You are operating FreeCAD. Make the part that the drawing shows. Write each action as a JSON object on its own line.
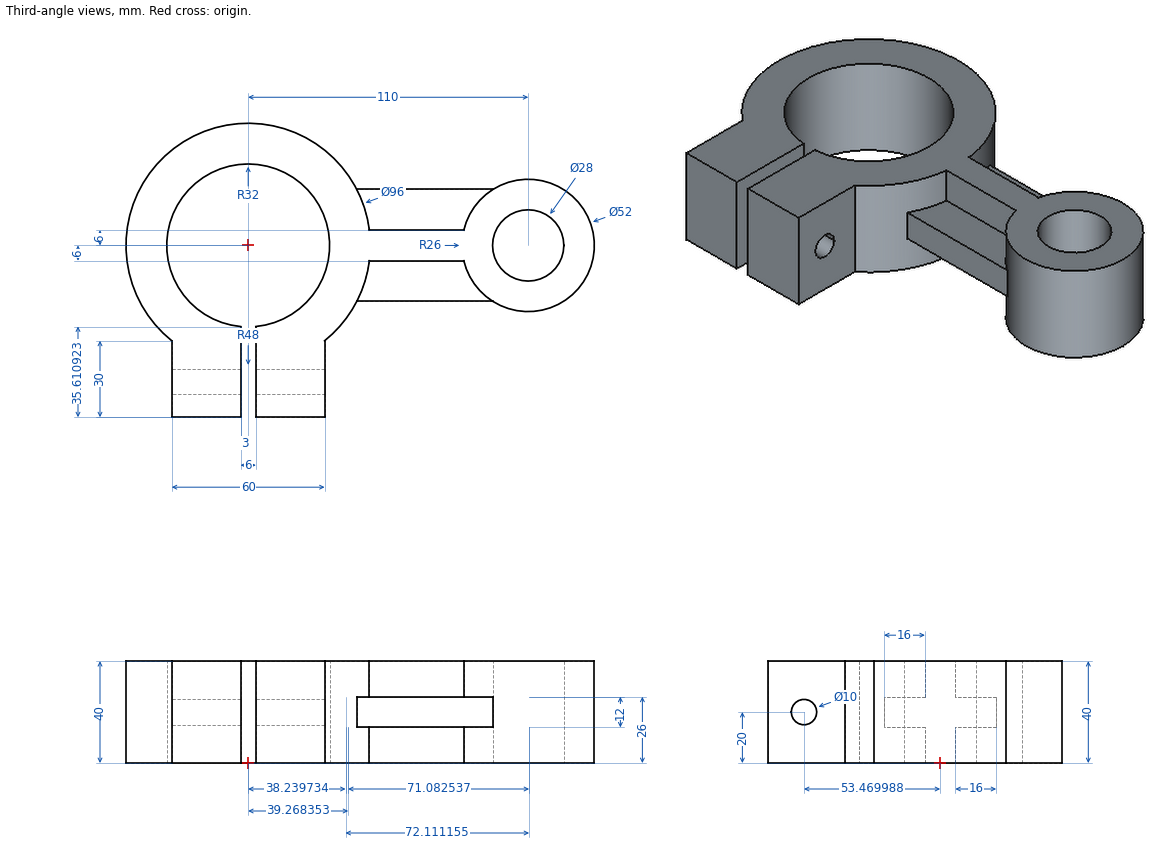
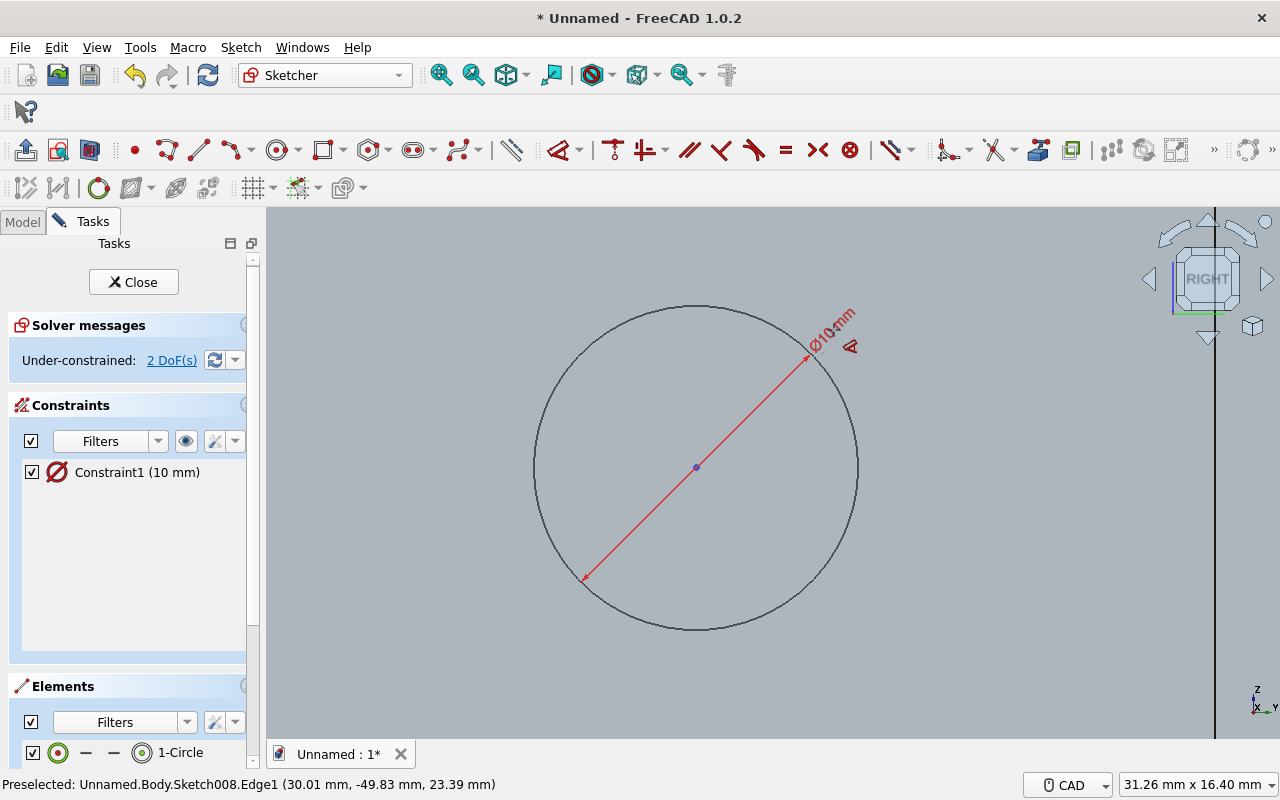
{"action": "left_click", "coordinate": [696, 468]}
{"action": "left_click", "coordinate": [662, 589]}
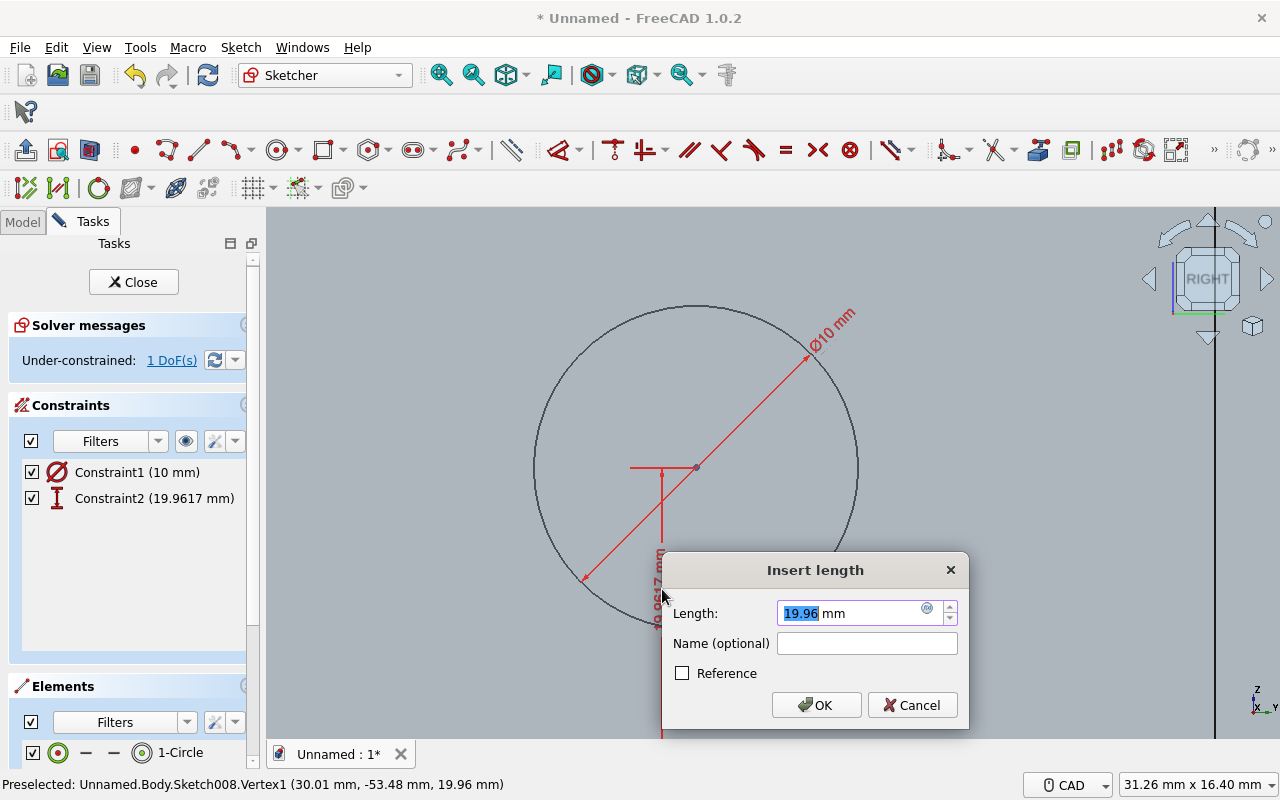
{"action": "type", "text": "20"}
{"action": "key", "text": "Return"}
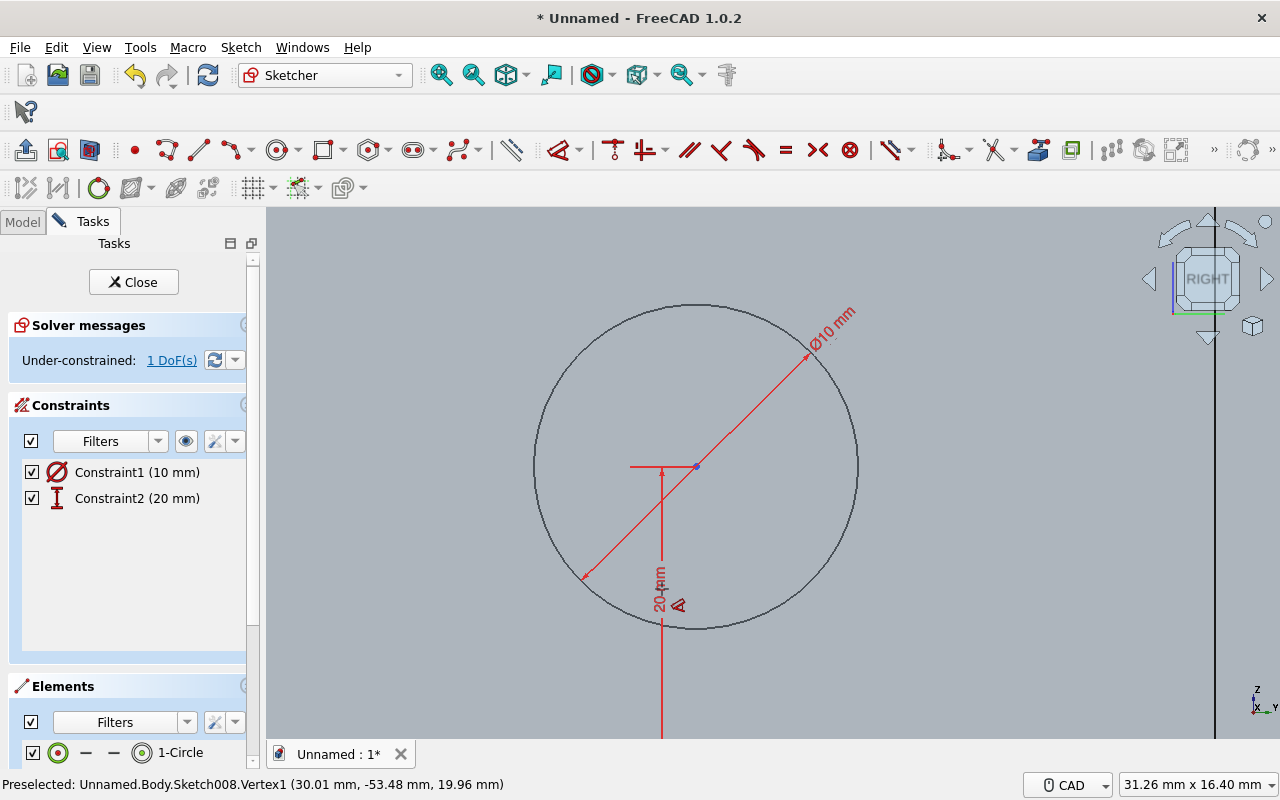
{"action": "left_click", "coordinate": [696, 467]}
{"action": "left_click", "coordinate": [906, 433]}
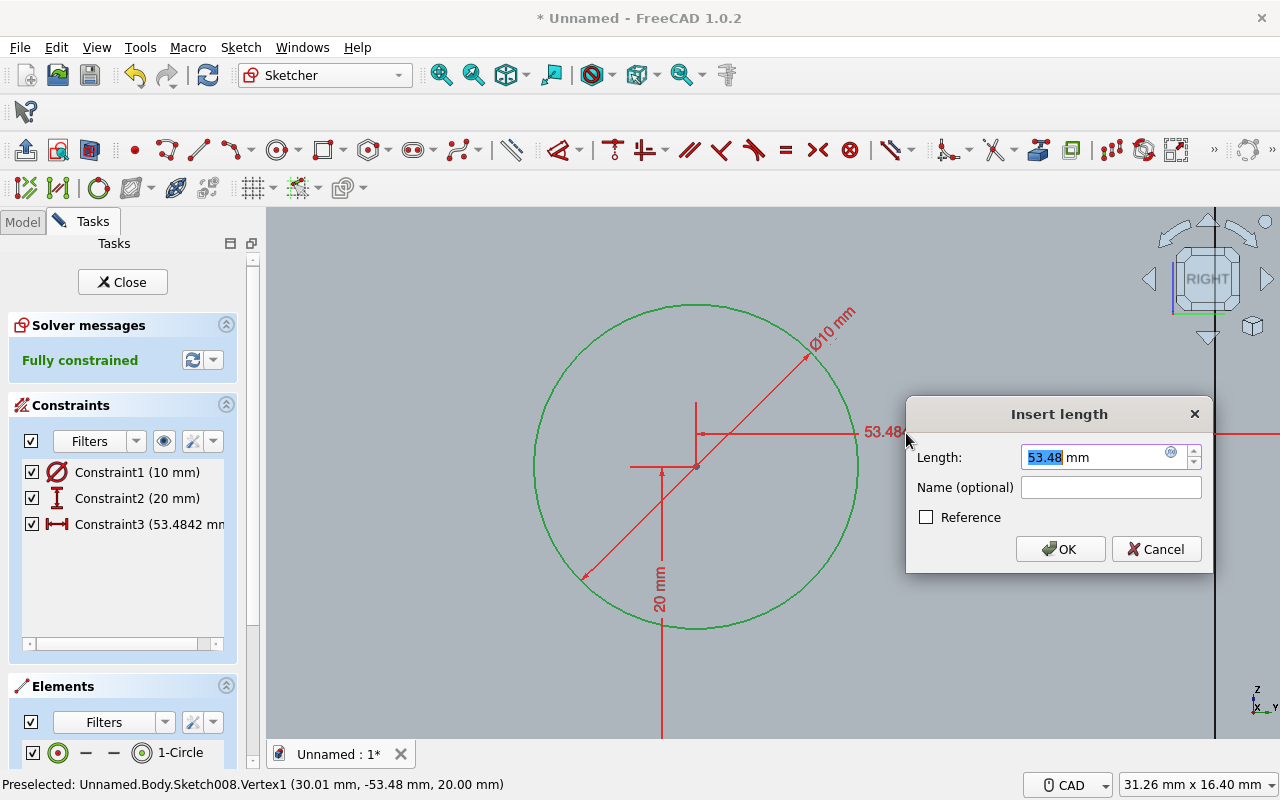
{"action": "type", "text": "53.469988"}
{"action": "key", "text": "Return"}
{"action": "key", "text": "Escape"}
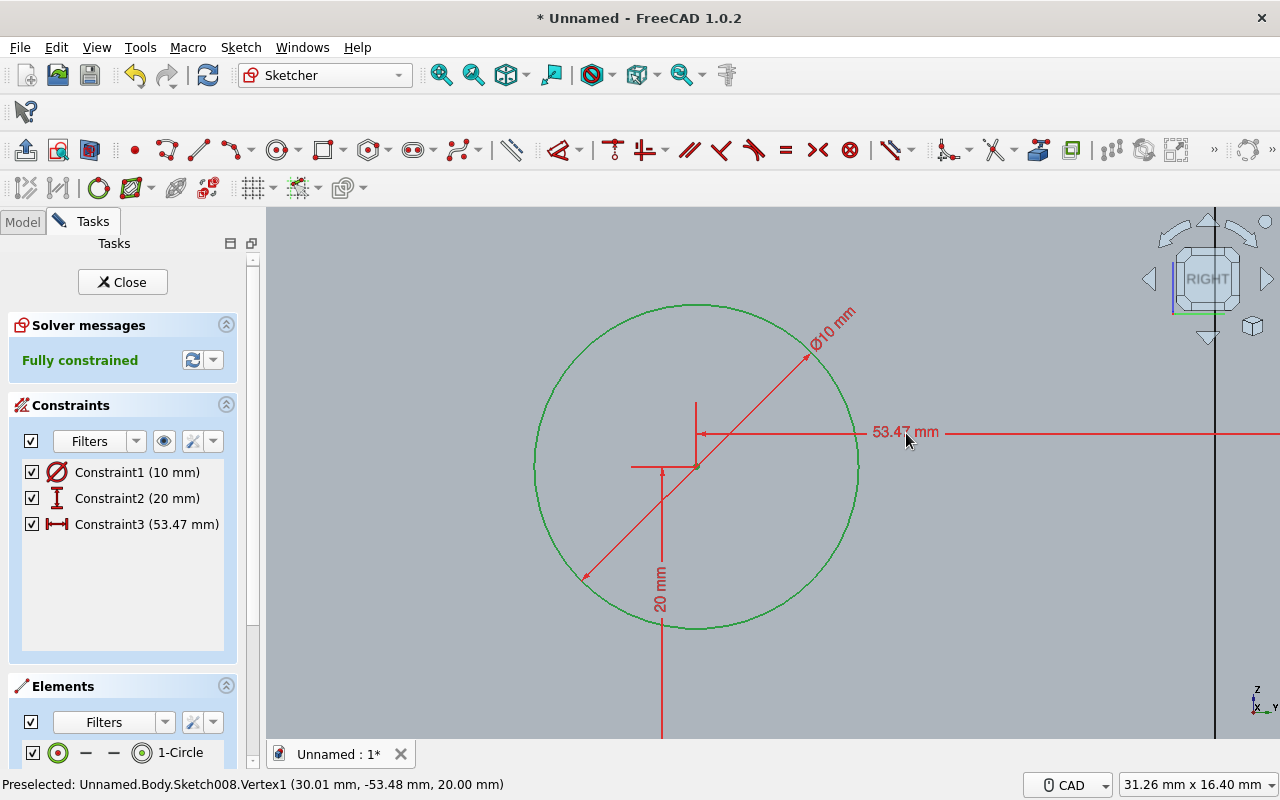
{"action": "left_click", "coordinate": [123, 282]}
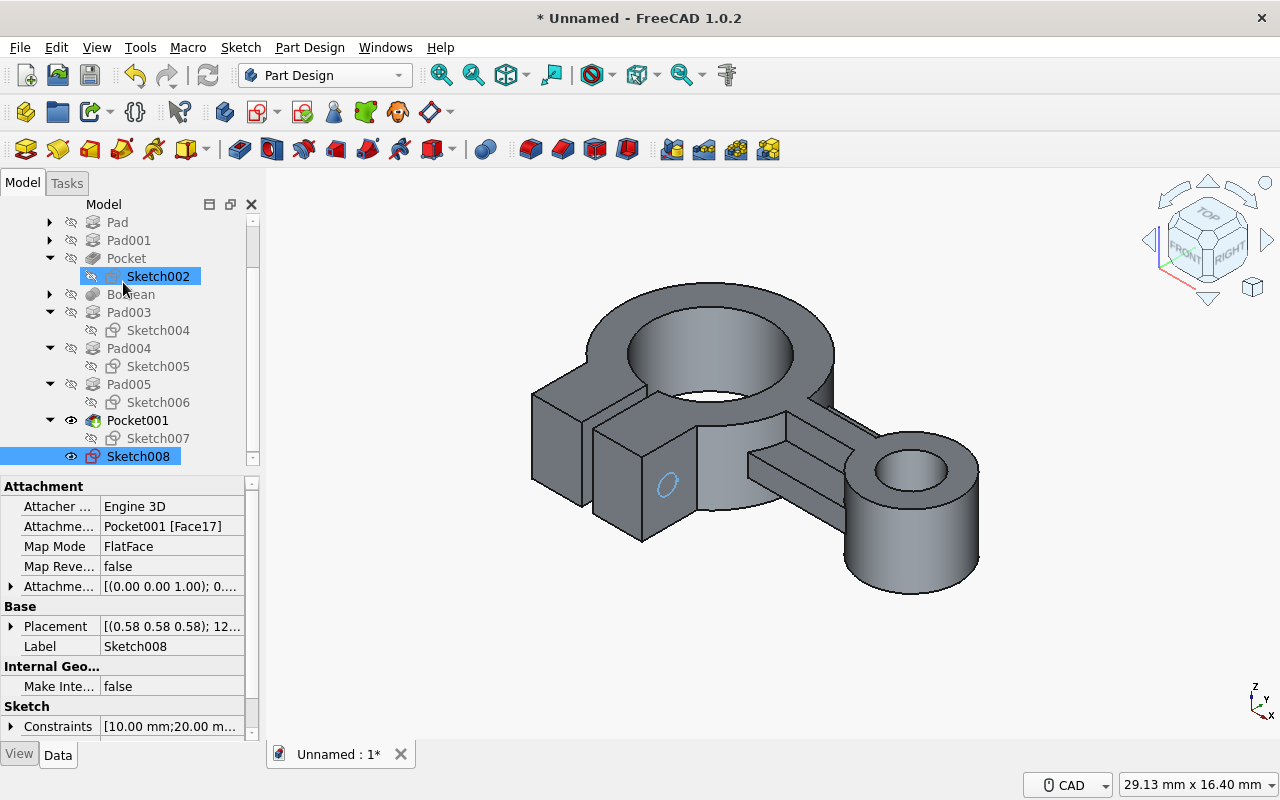
{"action": "left_click", "coordinate": [240, 150]}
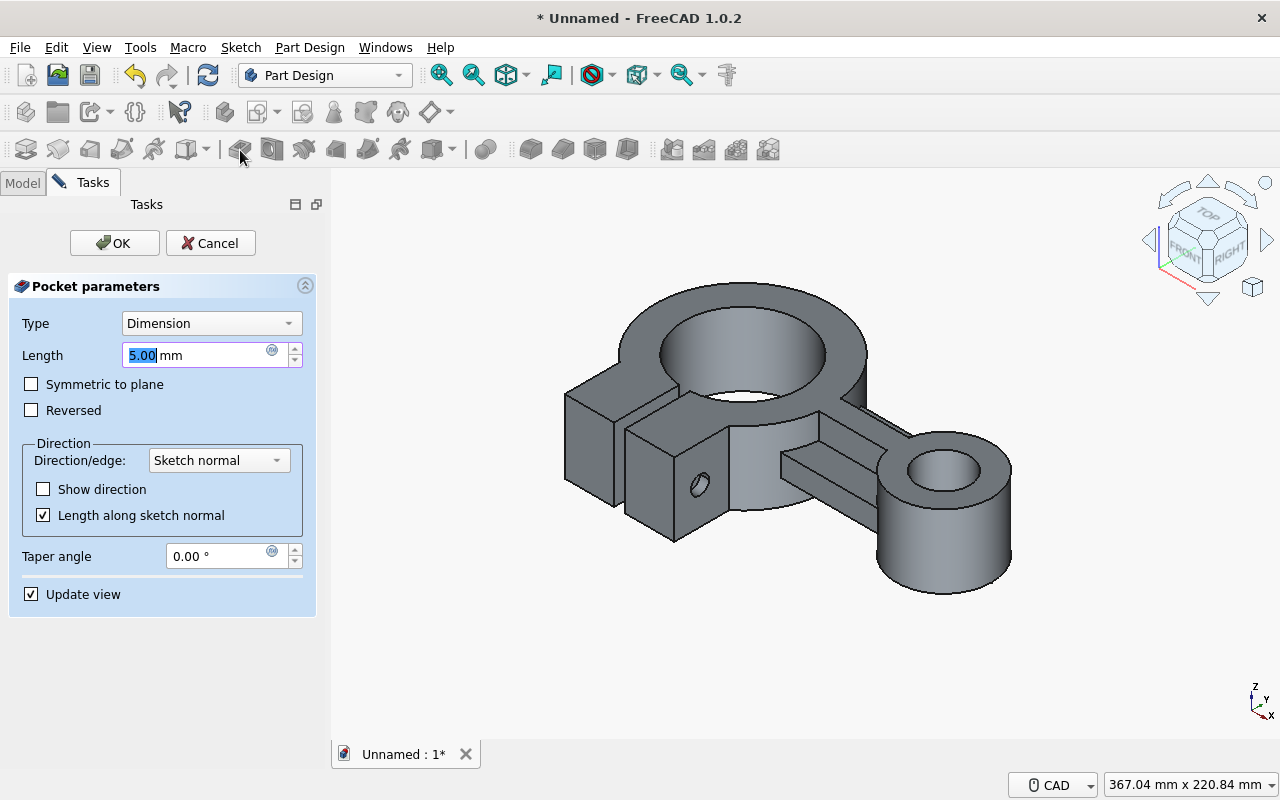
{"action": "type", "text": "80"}
{"action": "key", "text": "Tab"}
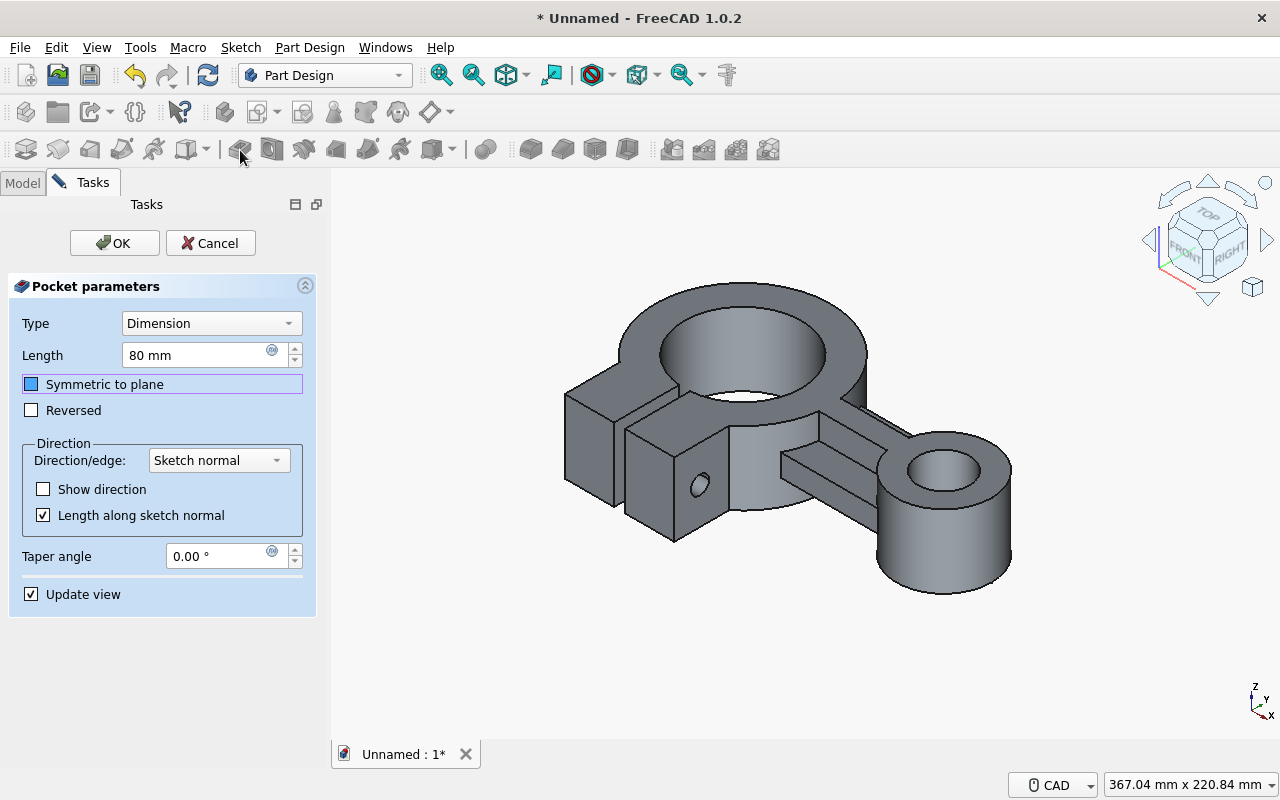
{"action": "left_click", "coordinate": [115, 243]}